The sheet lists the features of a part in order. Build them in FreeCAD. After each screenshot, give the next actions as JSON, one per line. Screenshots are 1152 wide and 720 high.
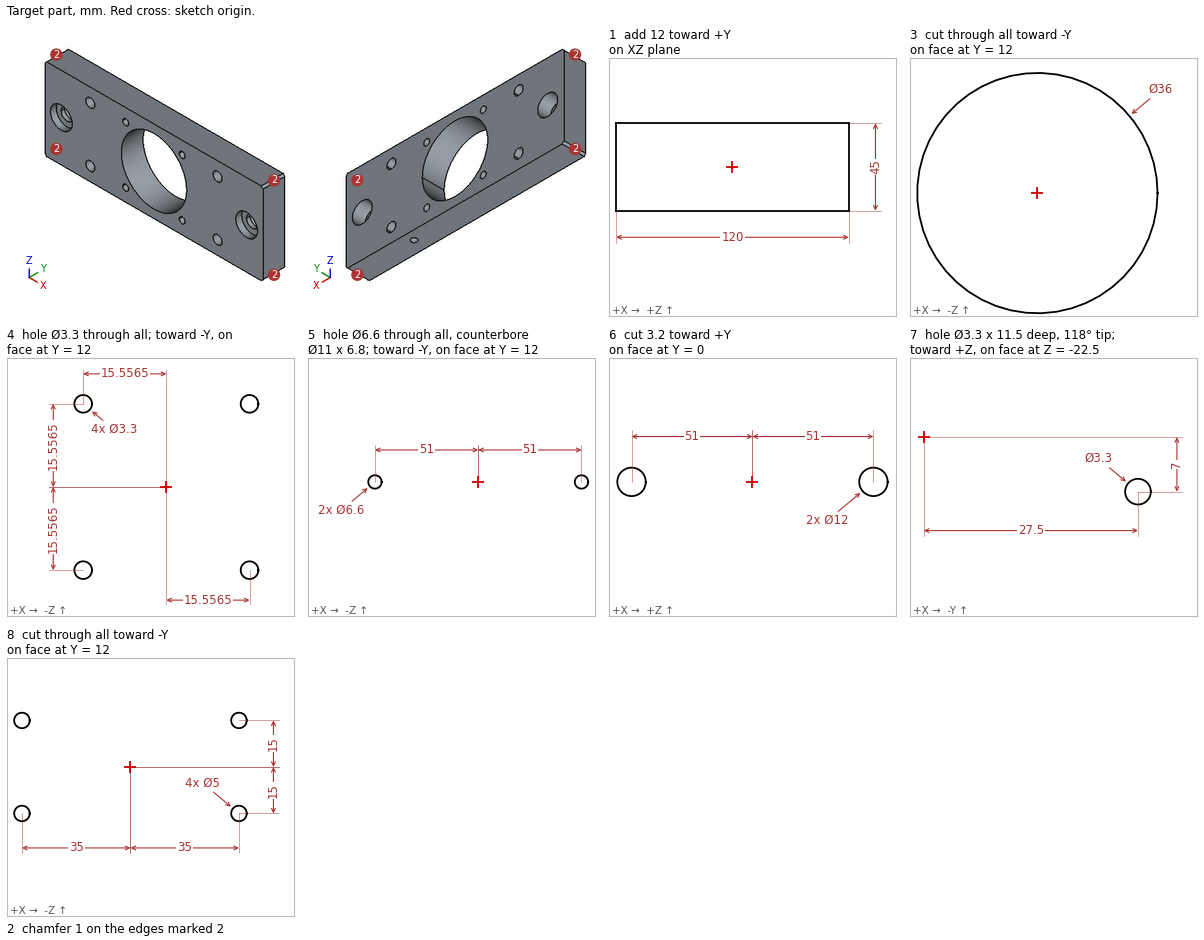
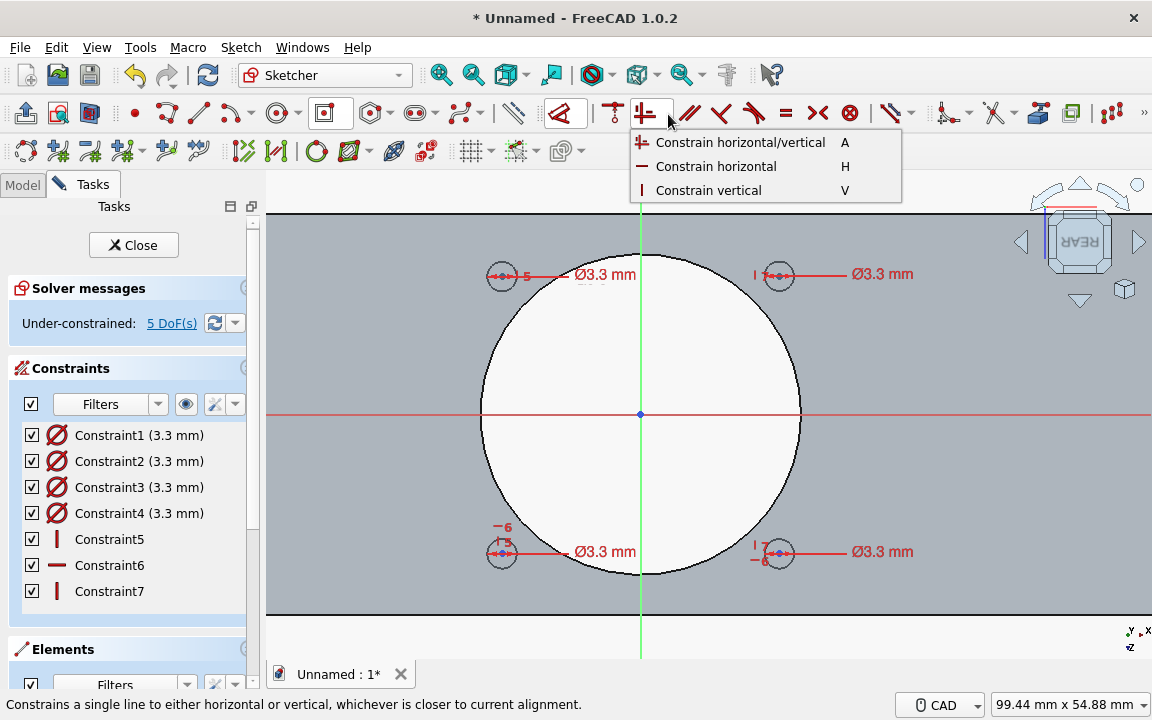
{"action": "left_click", "coordinate": [766, 166]}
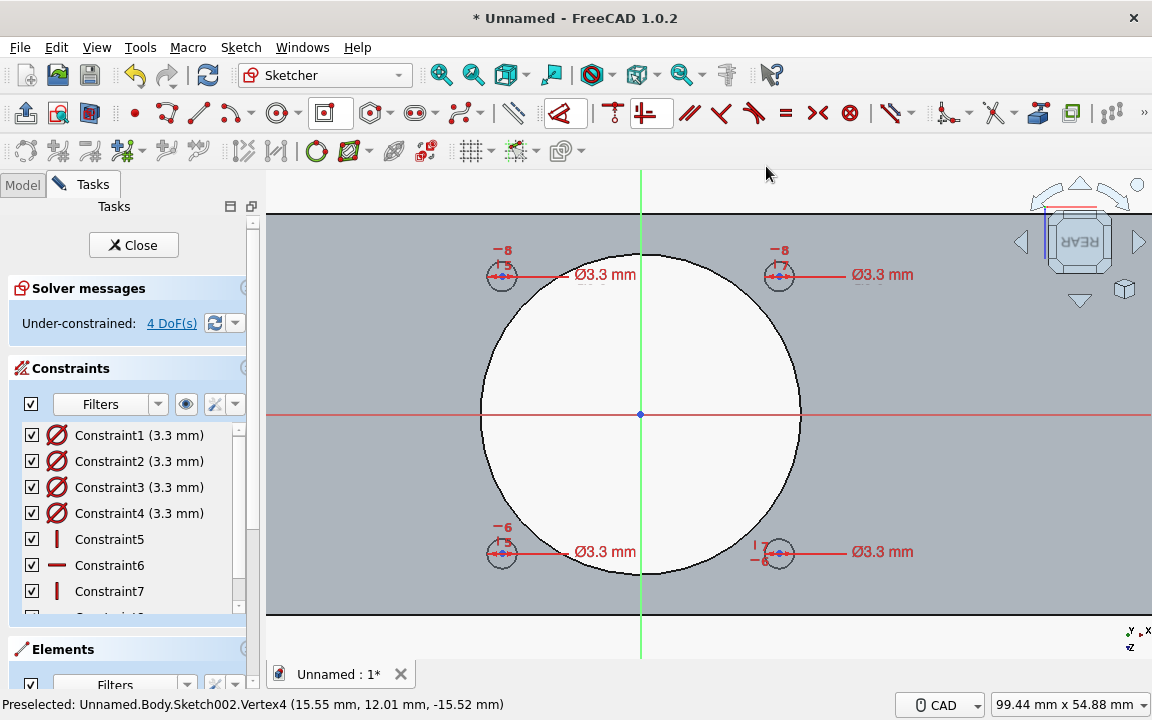
{"action": "left_click", "coordinate": [560, 114]}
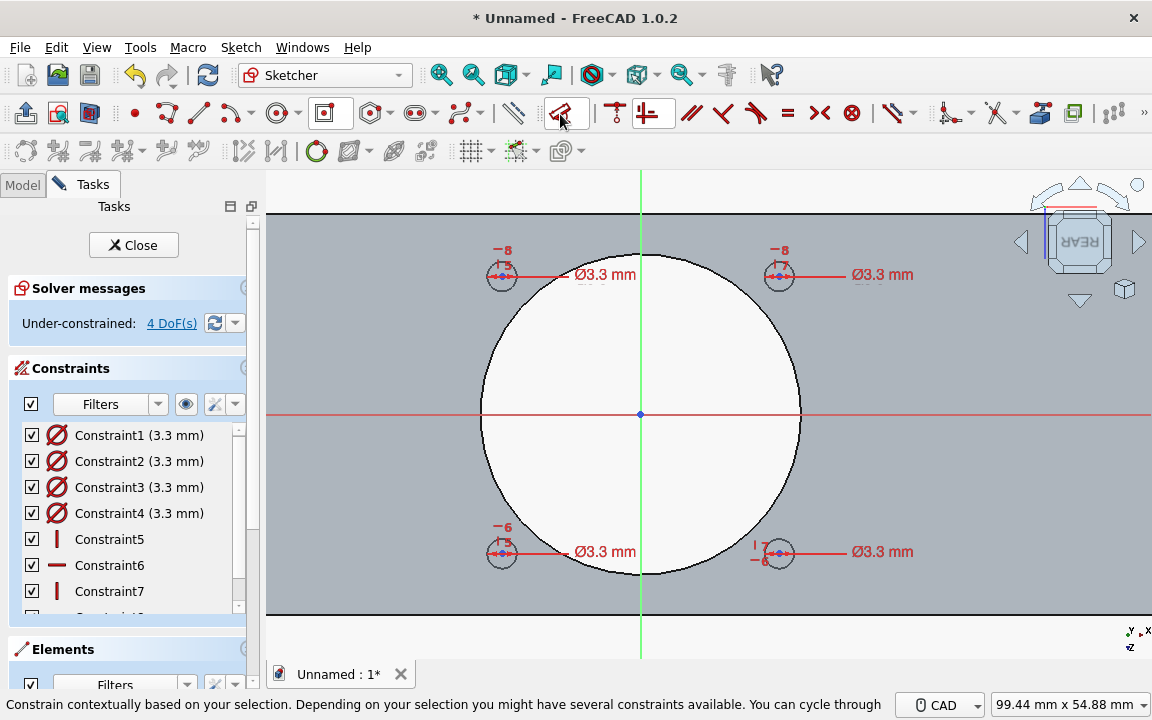
{"action": "left_click", "coordinate": [502, 277]}
{"action": "left_click", "coordinate": [571, 243]}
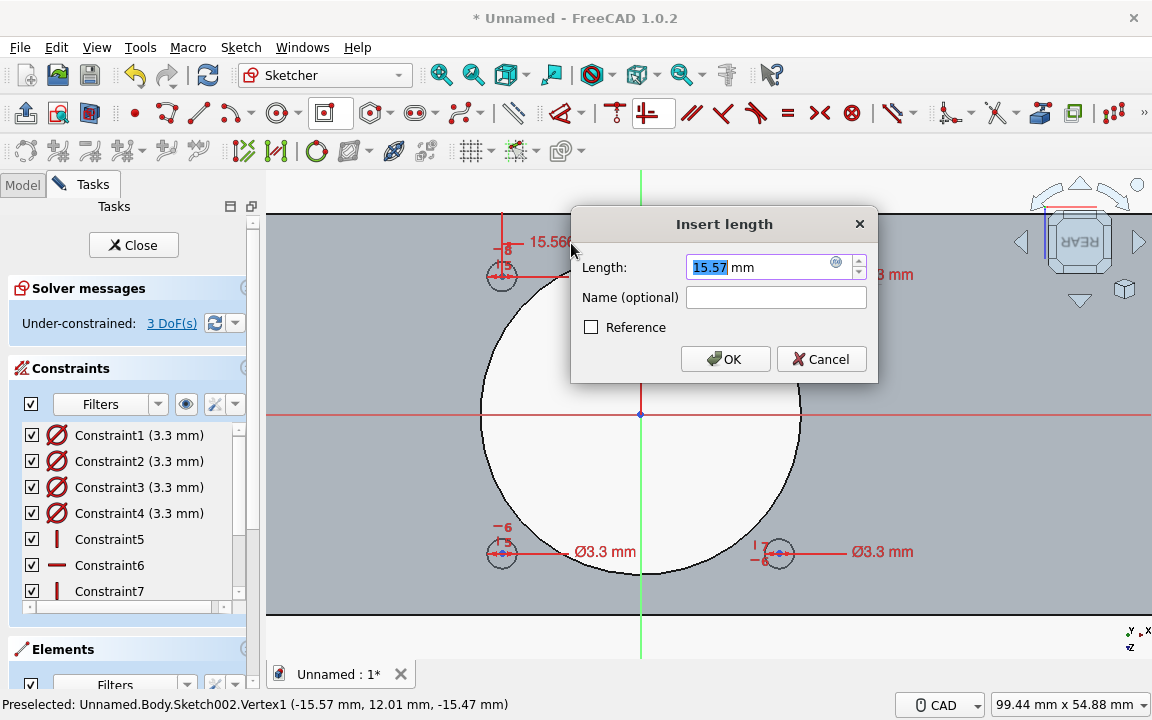
{"action": "type", "text": "15.5565"}
{"action": "key", "text": "Return"}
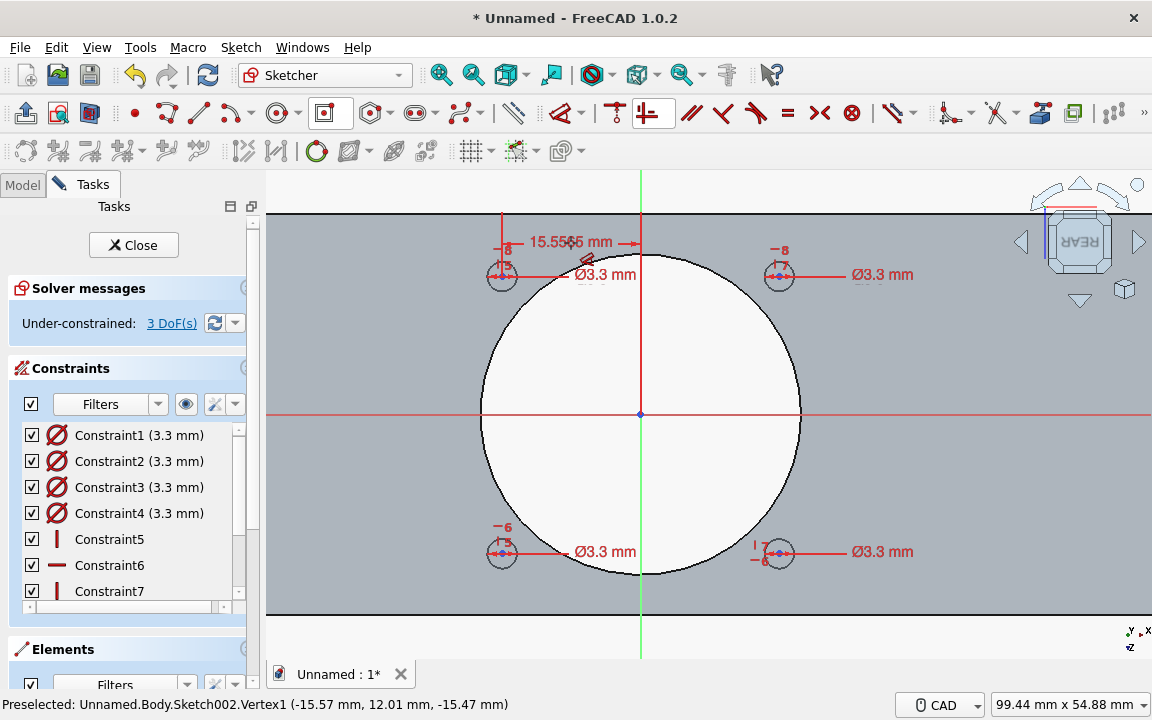
{"action": "left_click", "coordinate": [502, 277]}
{"action": "left_click", "coordinate": [468, 346]}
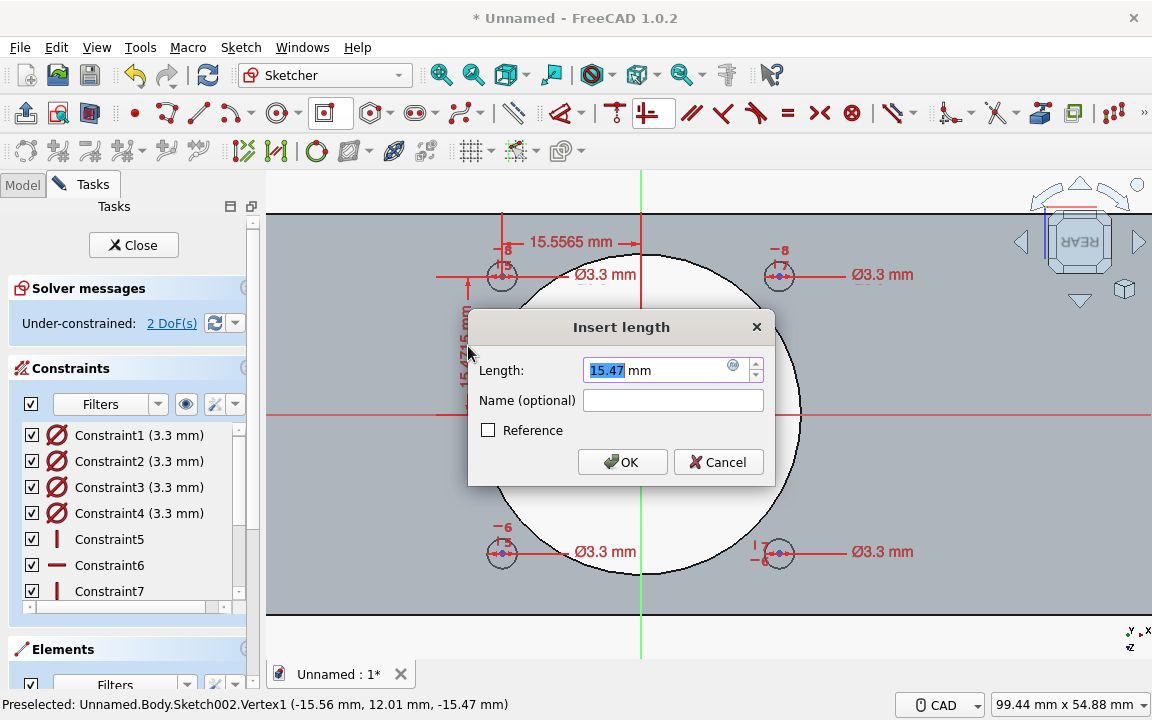
{"action": "type", "text": "15.5565"}
{"action": "key", "text": "Return"}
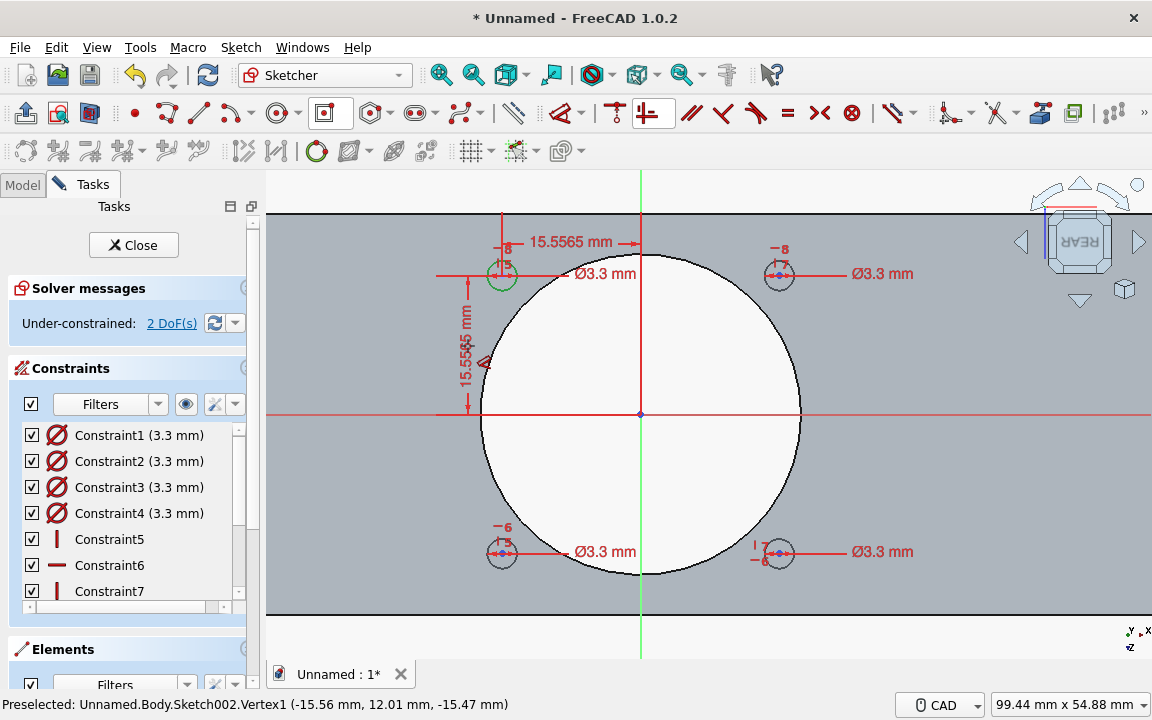
{"action": "left_click", "coordinate": [502, 554]}
{"action": "left_click", "coordinate": [468, 484]}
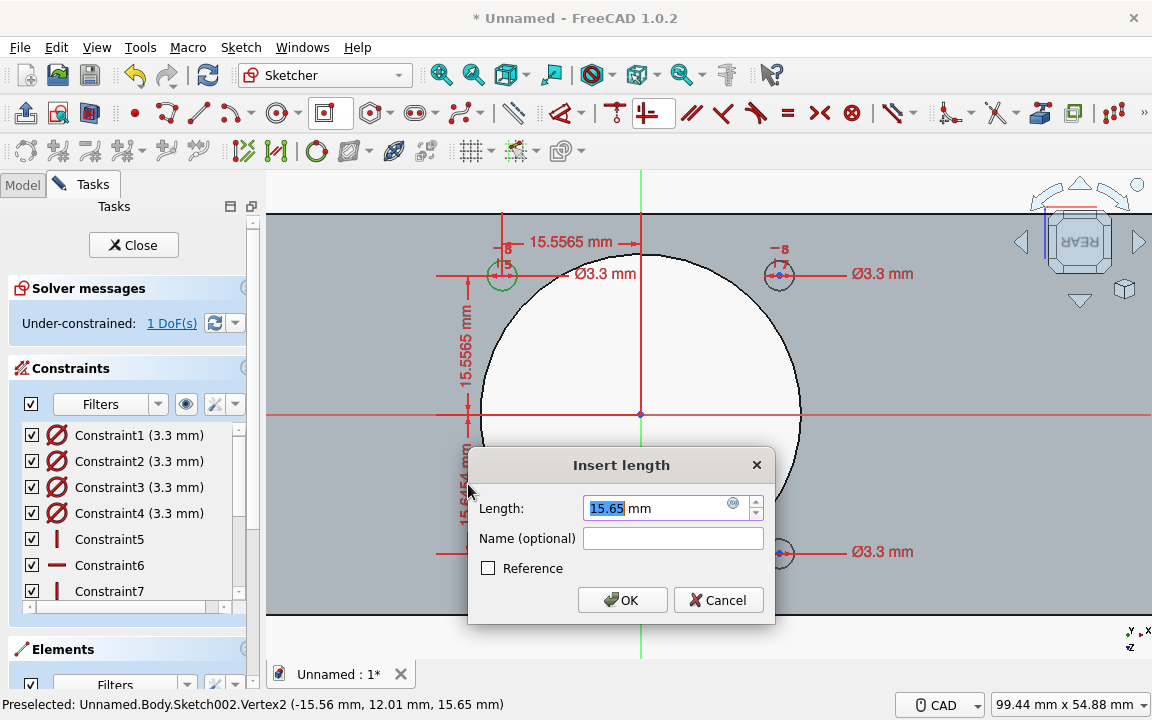
{"action": "type", "text": "15.5565"}
{"action": "key", "text": "Return"}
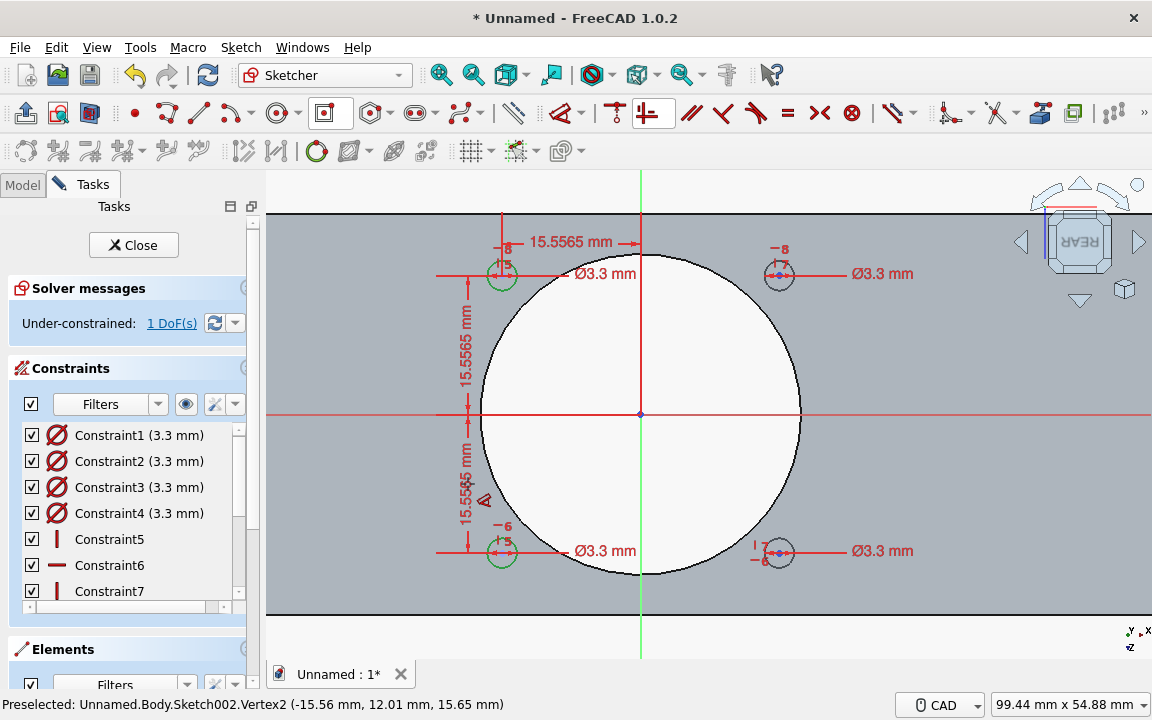
{"action": "left_click", "coordinate": [779, 553]}
{"action": "left_click", "coordinate": [710, 587]}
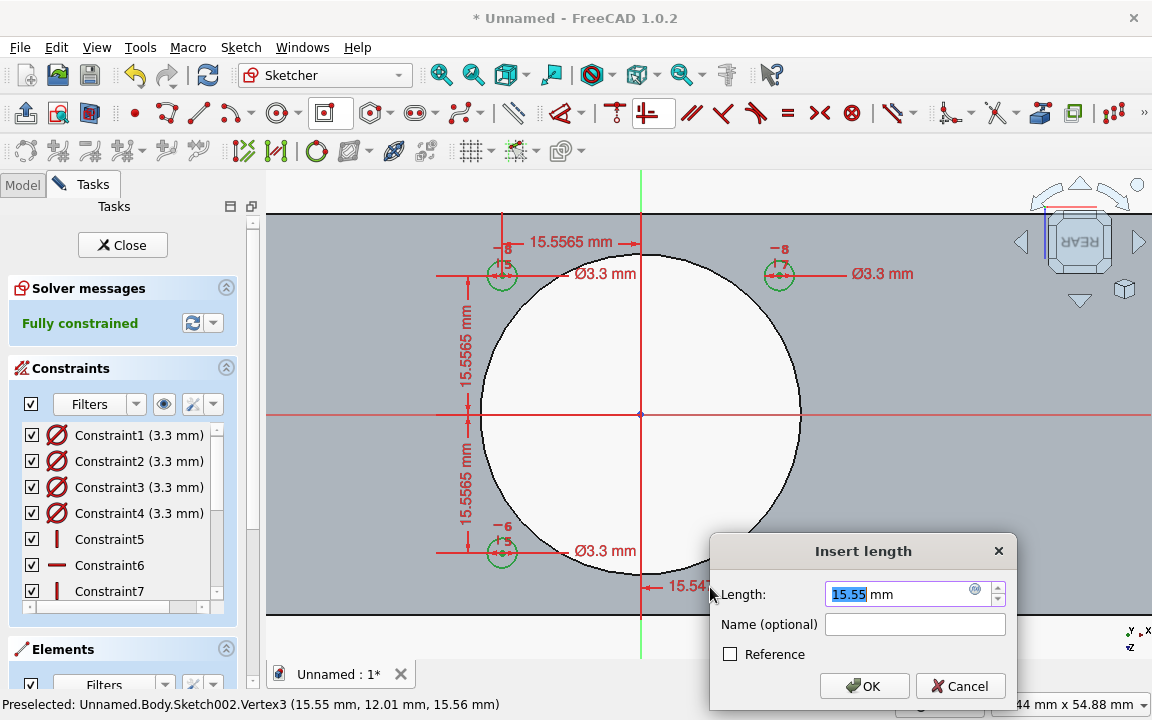
{"action": "type", "text": "15.5565"}
{"action": "key", "text": "Return"}
{"action": "key", "text": "Escape"}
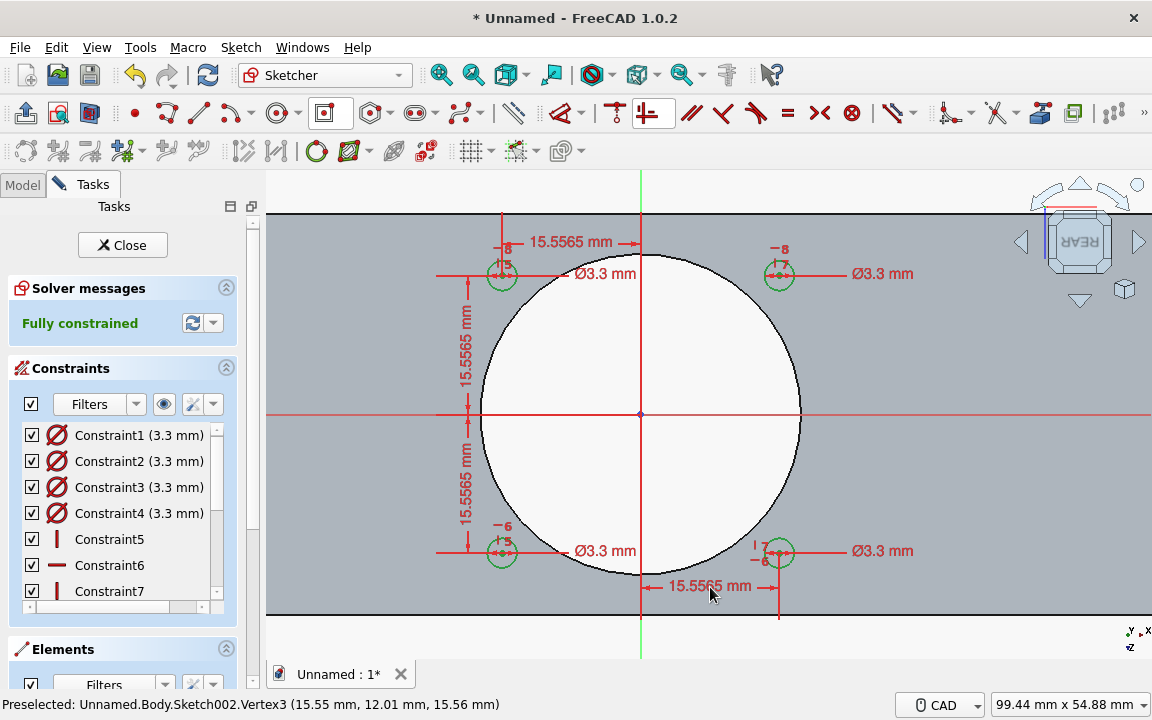
{"action": "left_click", "coordinate": [123, 245]}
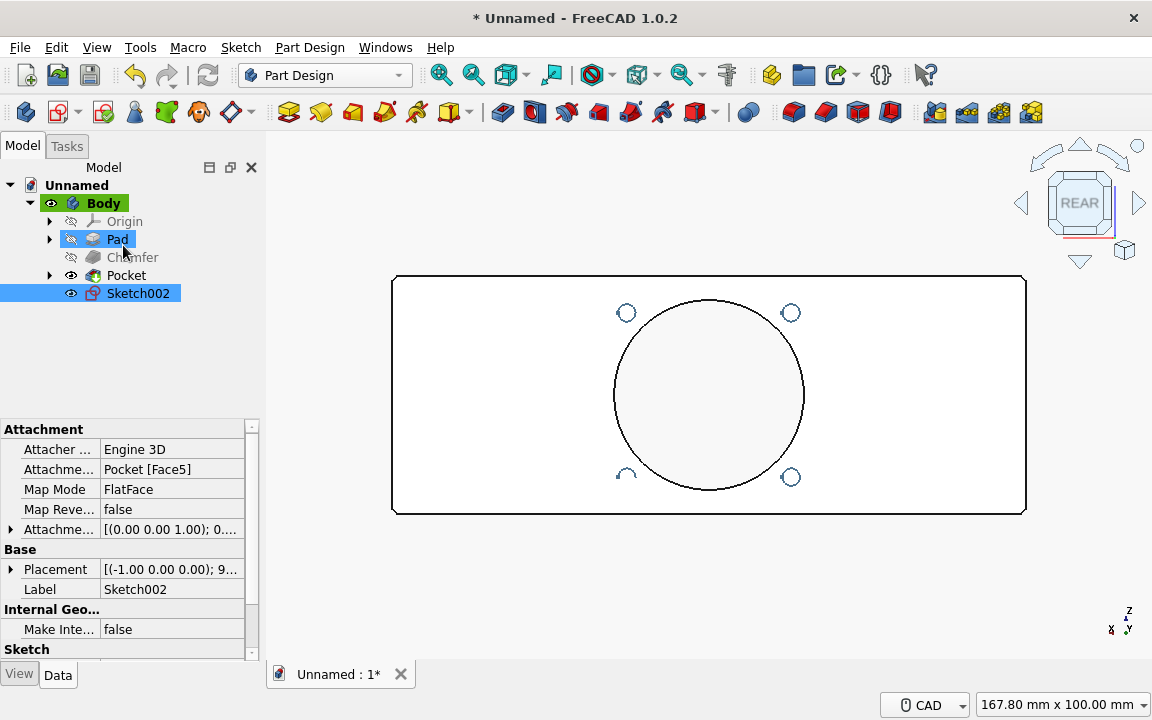
{"action": "left_click", "coordinate": [536, 112]}